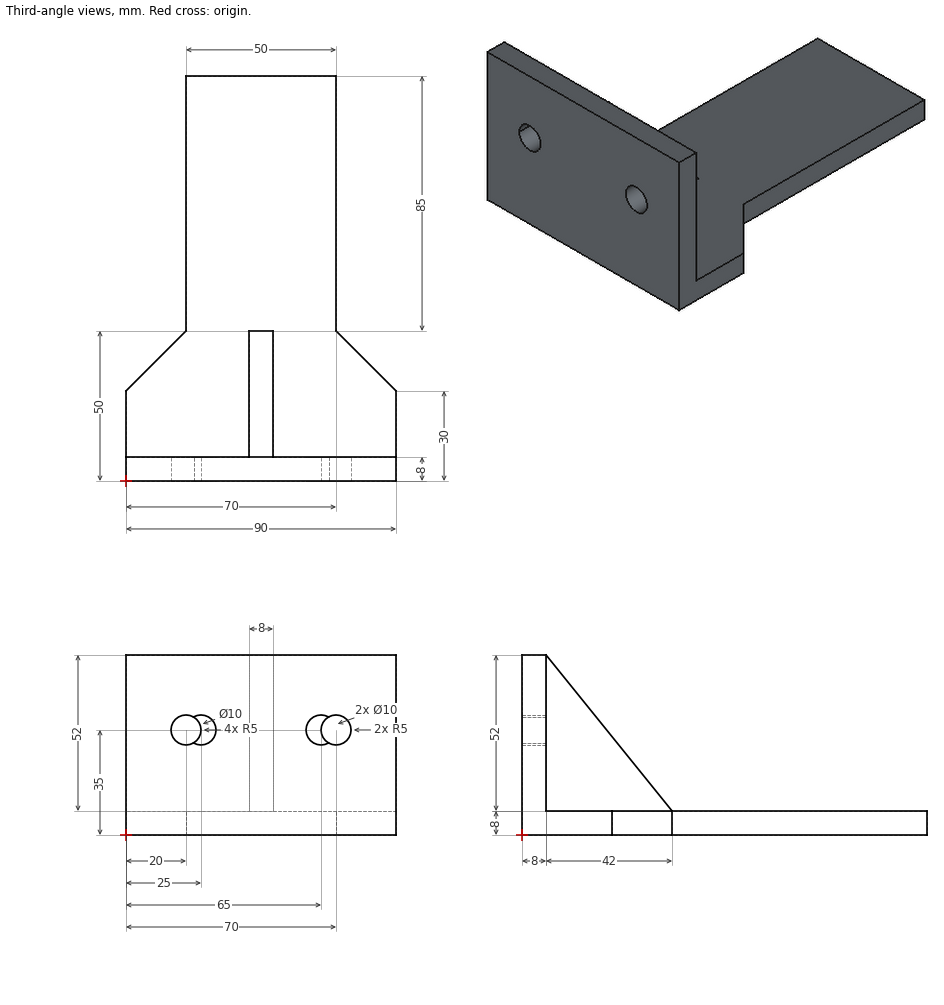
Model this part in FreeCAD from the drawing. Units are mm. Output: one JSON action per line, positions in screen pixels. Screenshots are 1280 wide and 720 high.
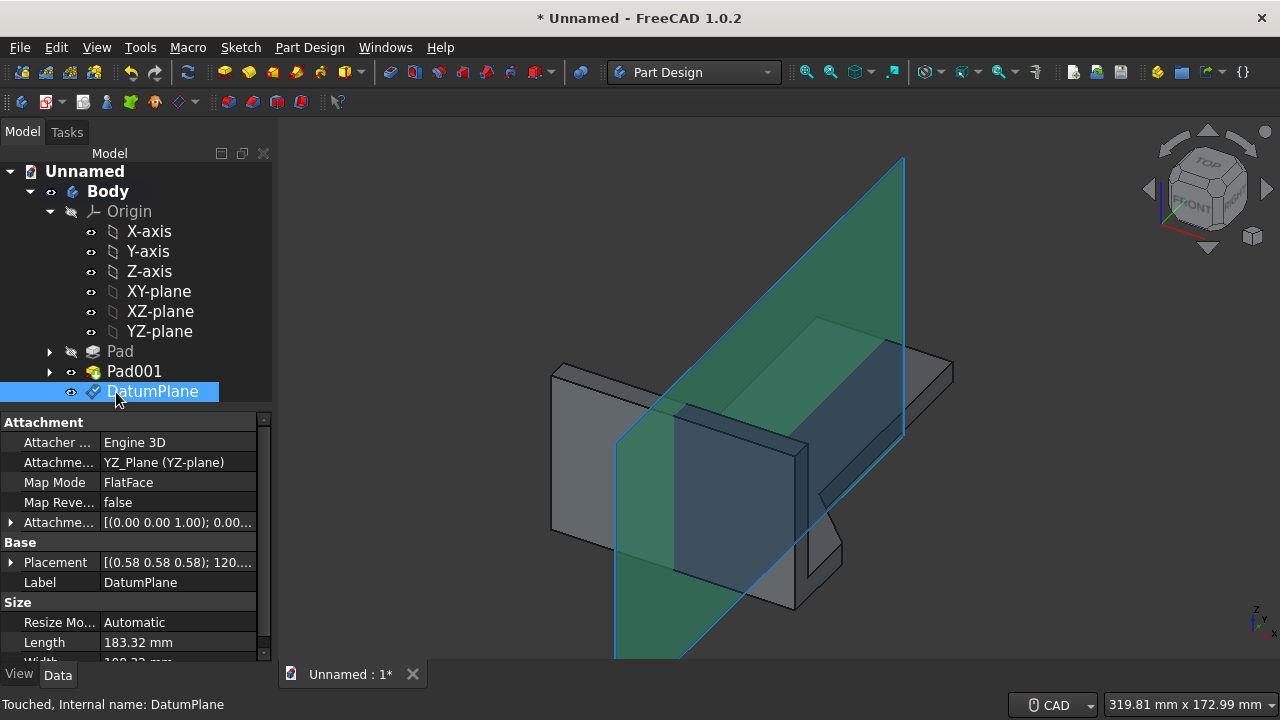
{"action": "left_click", "coordinate": [46, 102]}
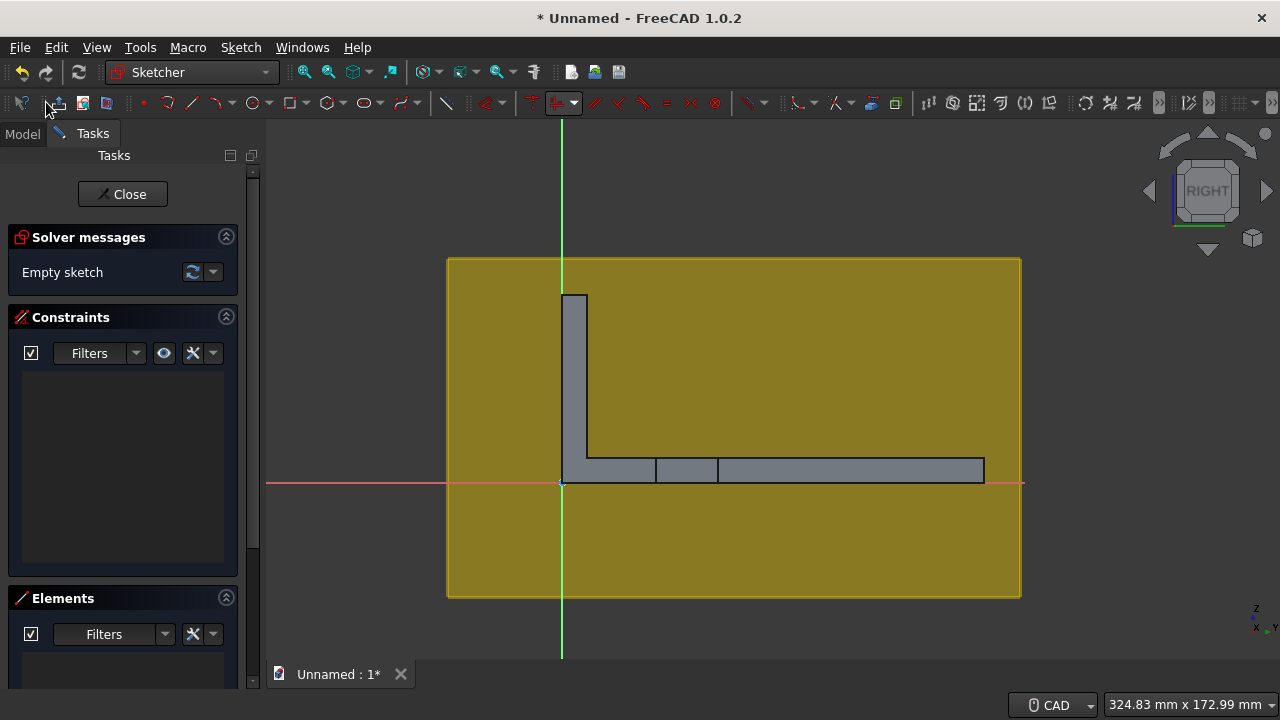
{"action": "left_click", "coordinate": [108, 104]}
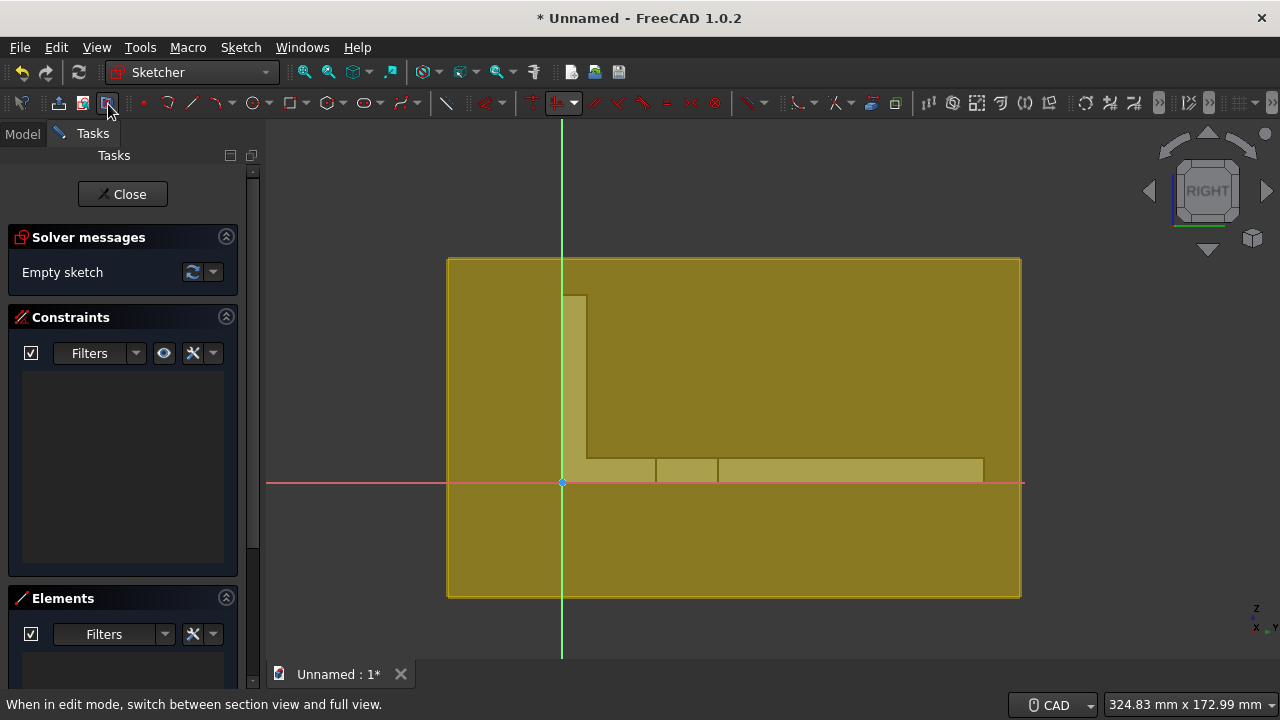
{"action": "scroll", "coordinate": [562, 389], "scroll_direction": "up", "scroll_amount": 3}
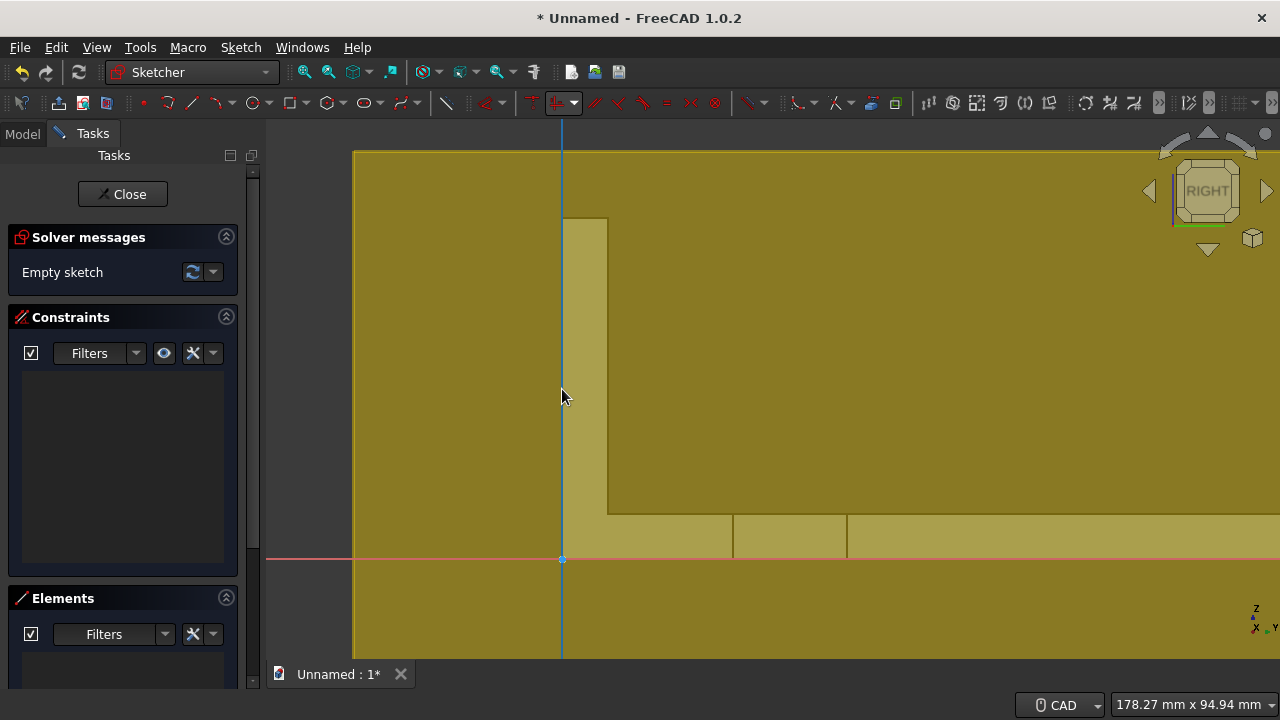
{"action": "left_click", "coordinate": [168, 104]}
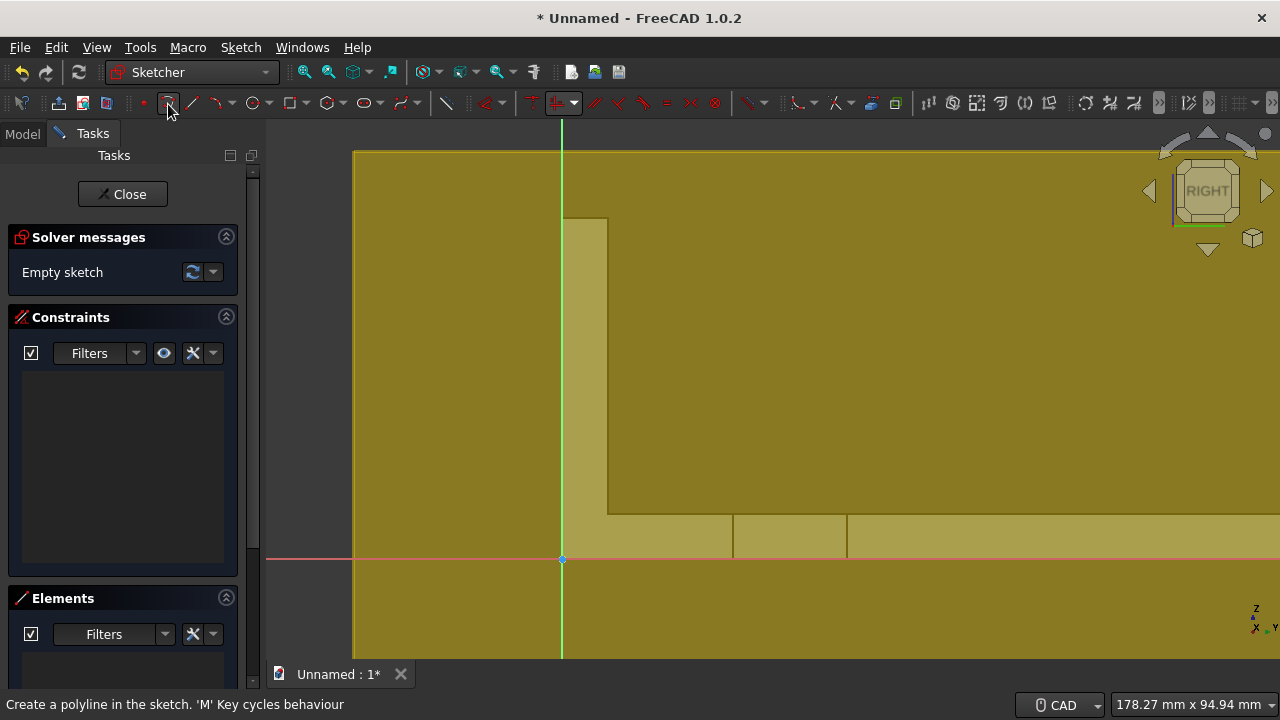
{"action": "left_click", "coordinate": [608, 514]}
{"action": "left_click", "coordinate": [847, 514]}
{"action": "left_click", "coordinate": [608, 218]}
{"action": "left_click", "coordinate": [608, 515]}
{"action": "key", "text": "Escape"}
{"action": "key", "text": "Escape"}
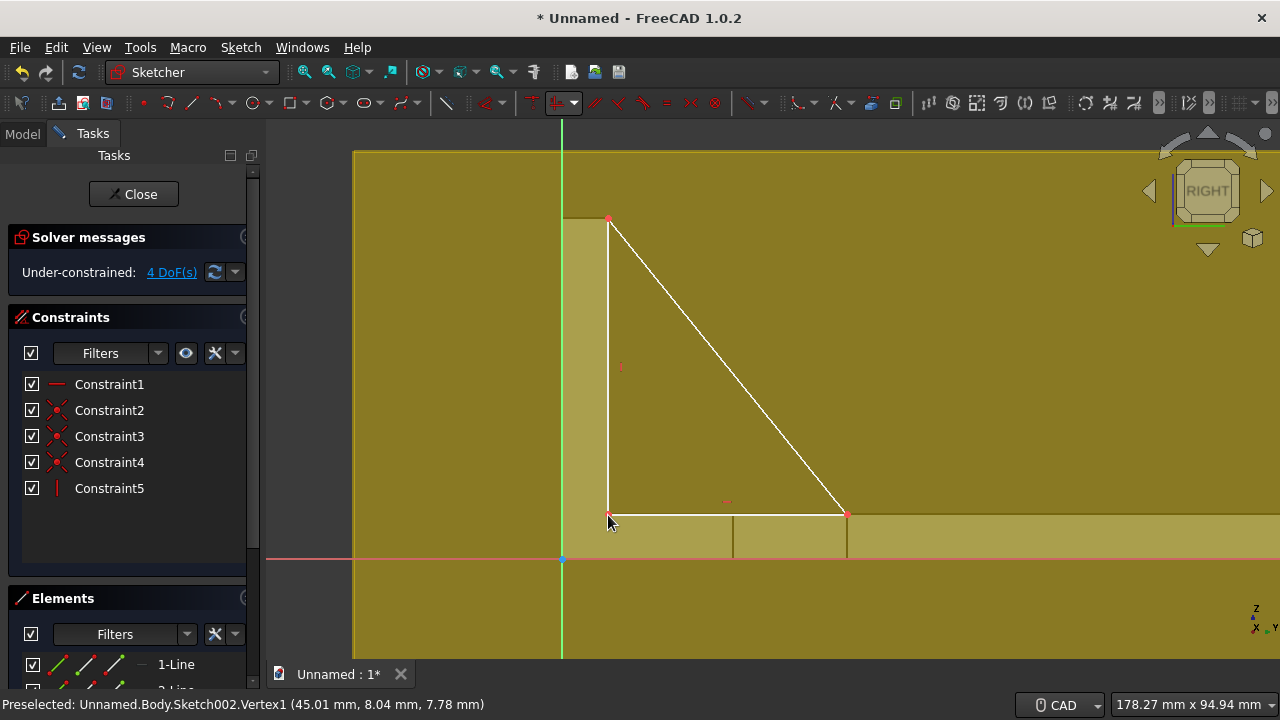
{"action": "left_click", "coordinate": [486, 104]}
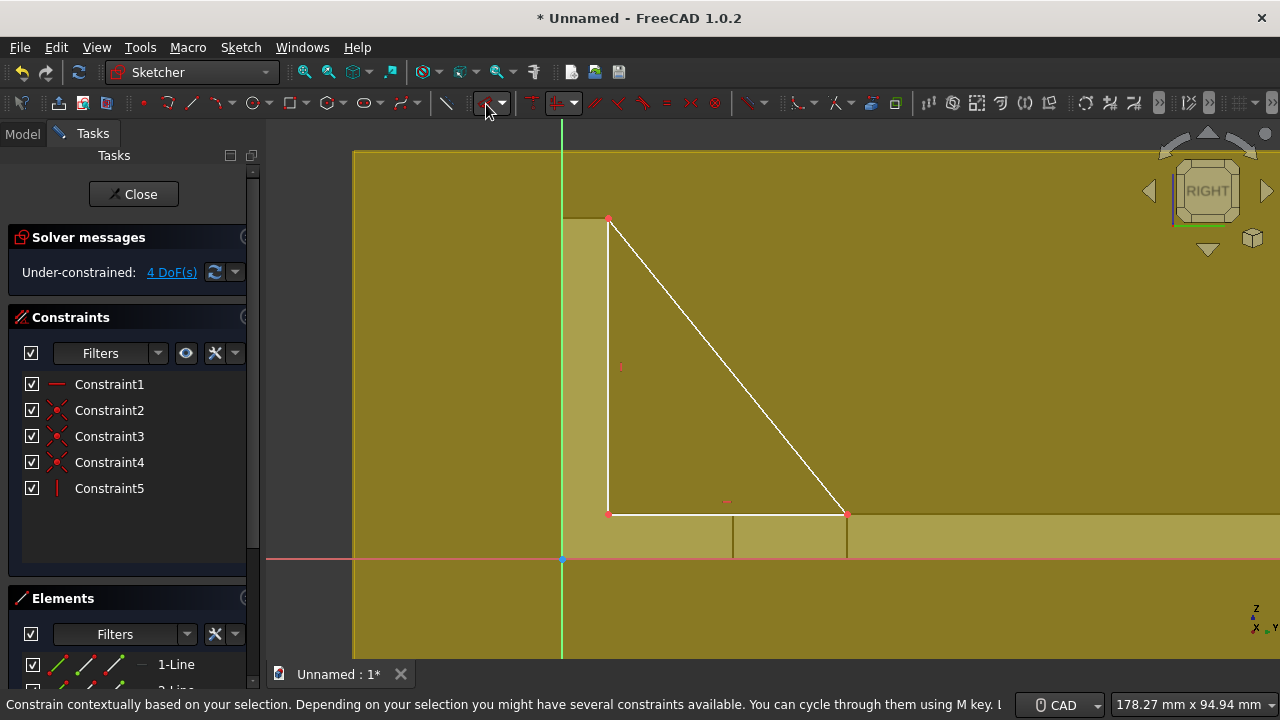
{"action": "left_click", "coordinate": [680, 515]}
{"action": "left_click", "coordinate": [727, 481]}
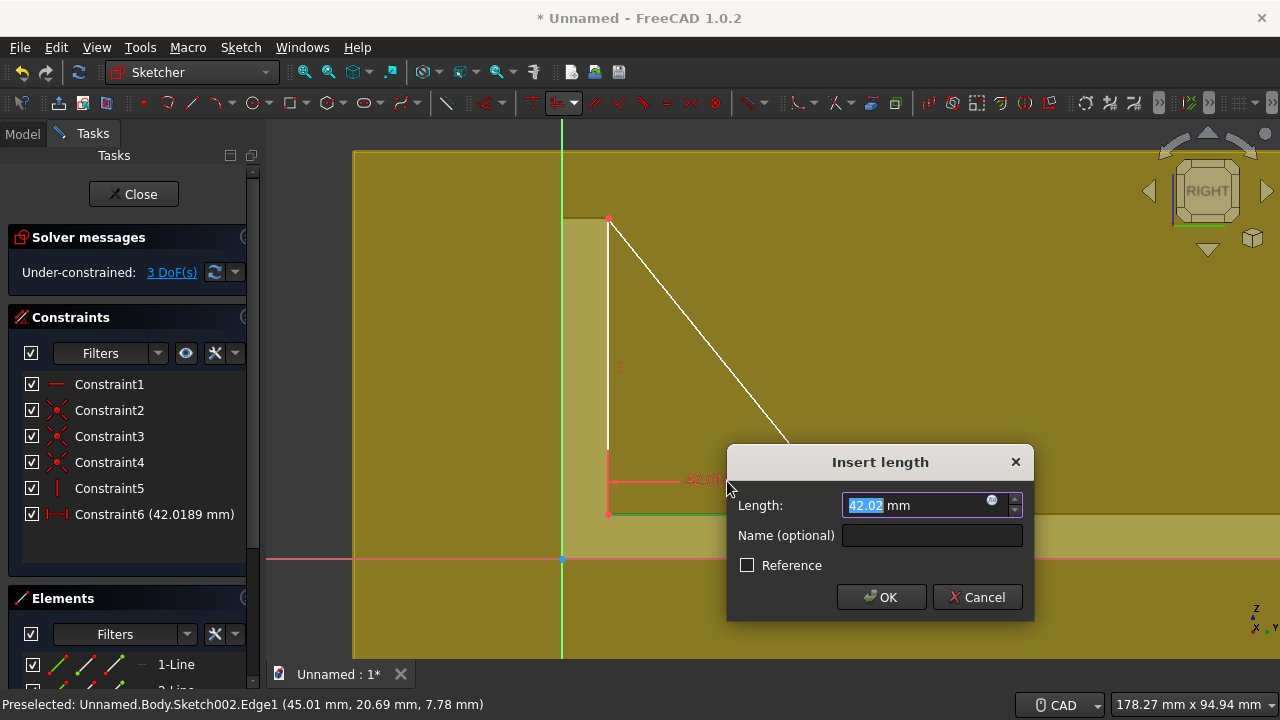
{"action": "type", "text": "42"}
{"action": "key", "text": "Return"}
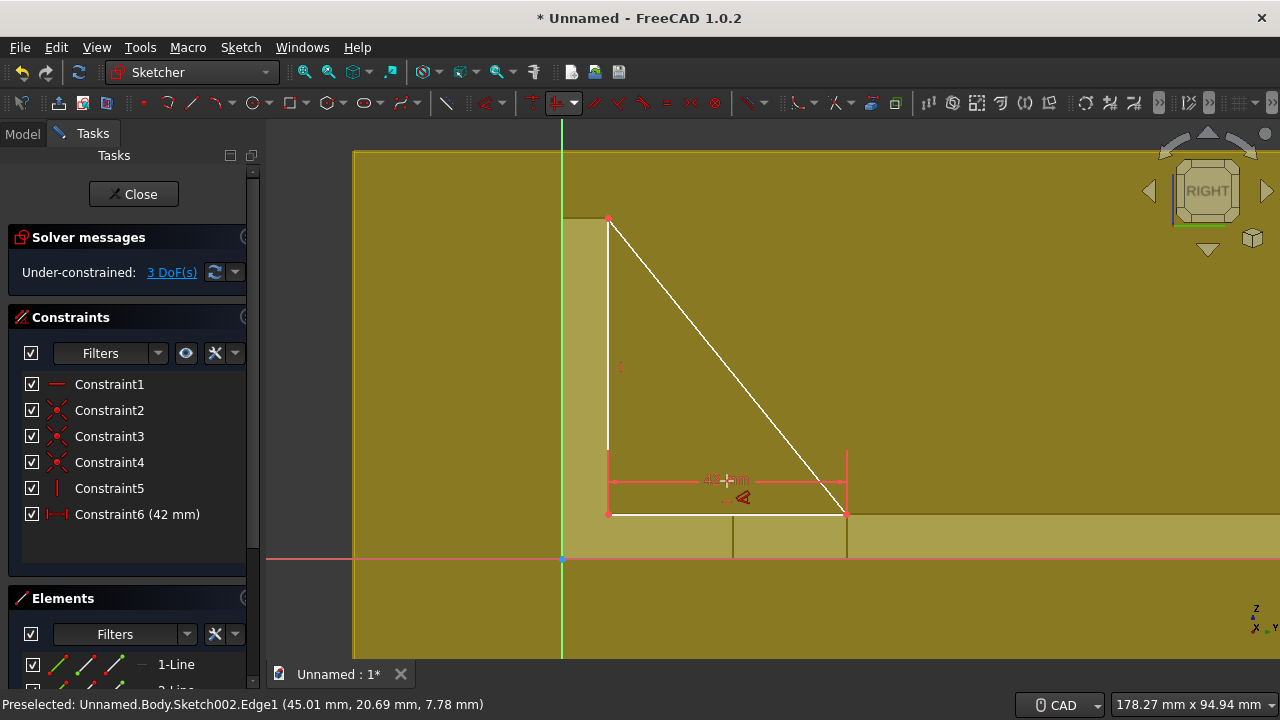
{"action": "left_click", "coordinate": [608, 308]}
{"action": "left_click", "coordinate": [642, 367]}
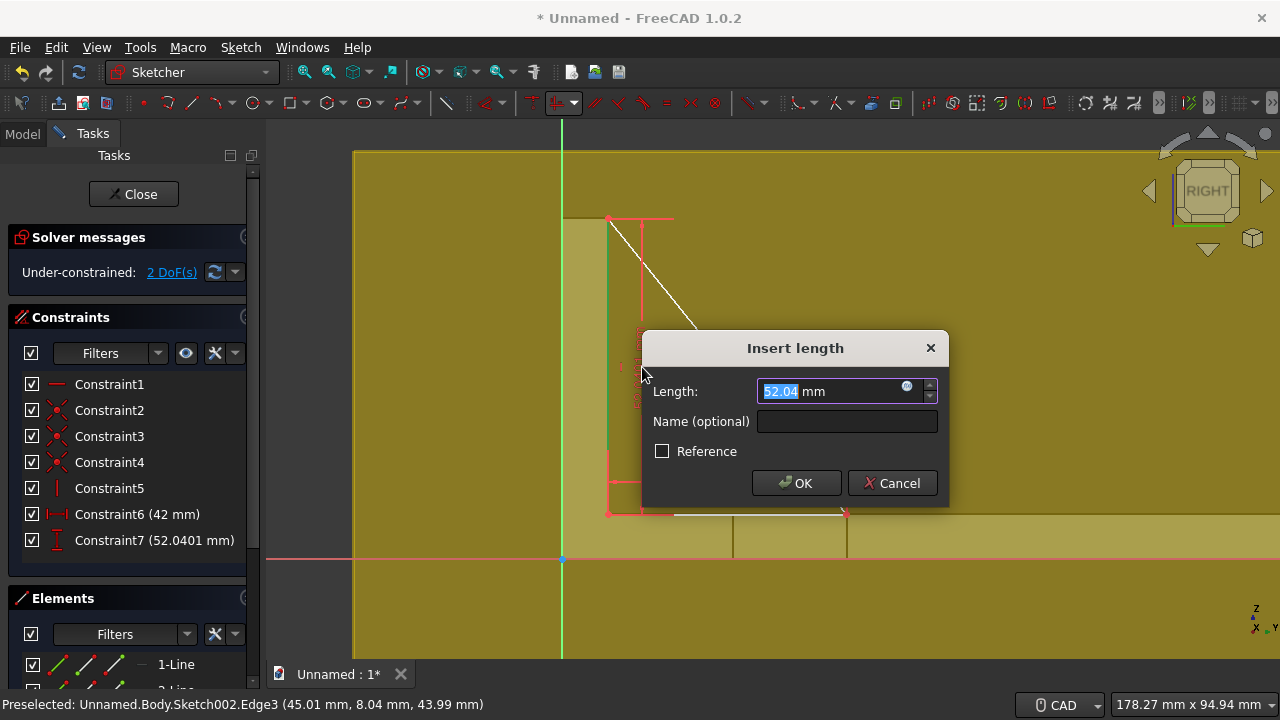
{"action": "type", "text": "52"}
{"action": "key", "text": "Return"}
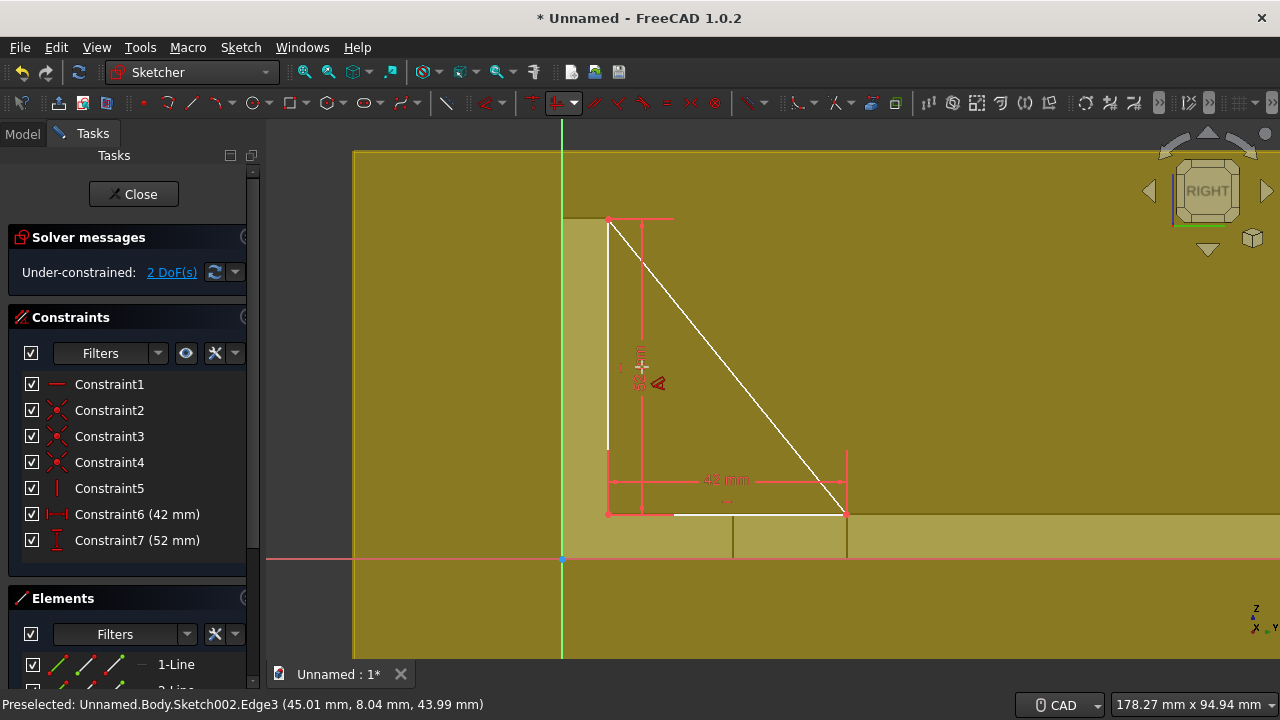
{"action": "left_click", "coordinate": [608, 515]}
{"action": "left_click", "coordinate": [585, 593]}